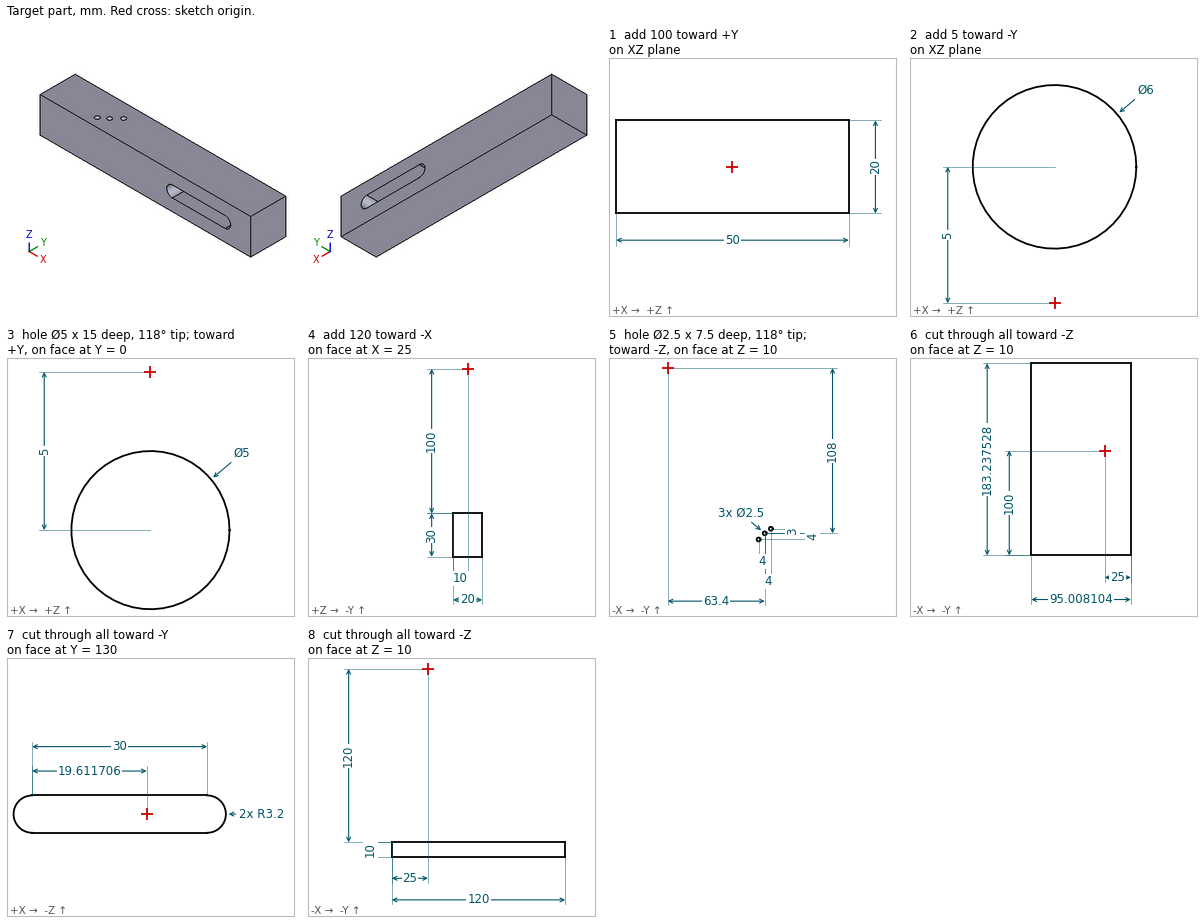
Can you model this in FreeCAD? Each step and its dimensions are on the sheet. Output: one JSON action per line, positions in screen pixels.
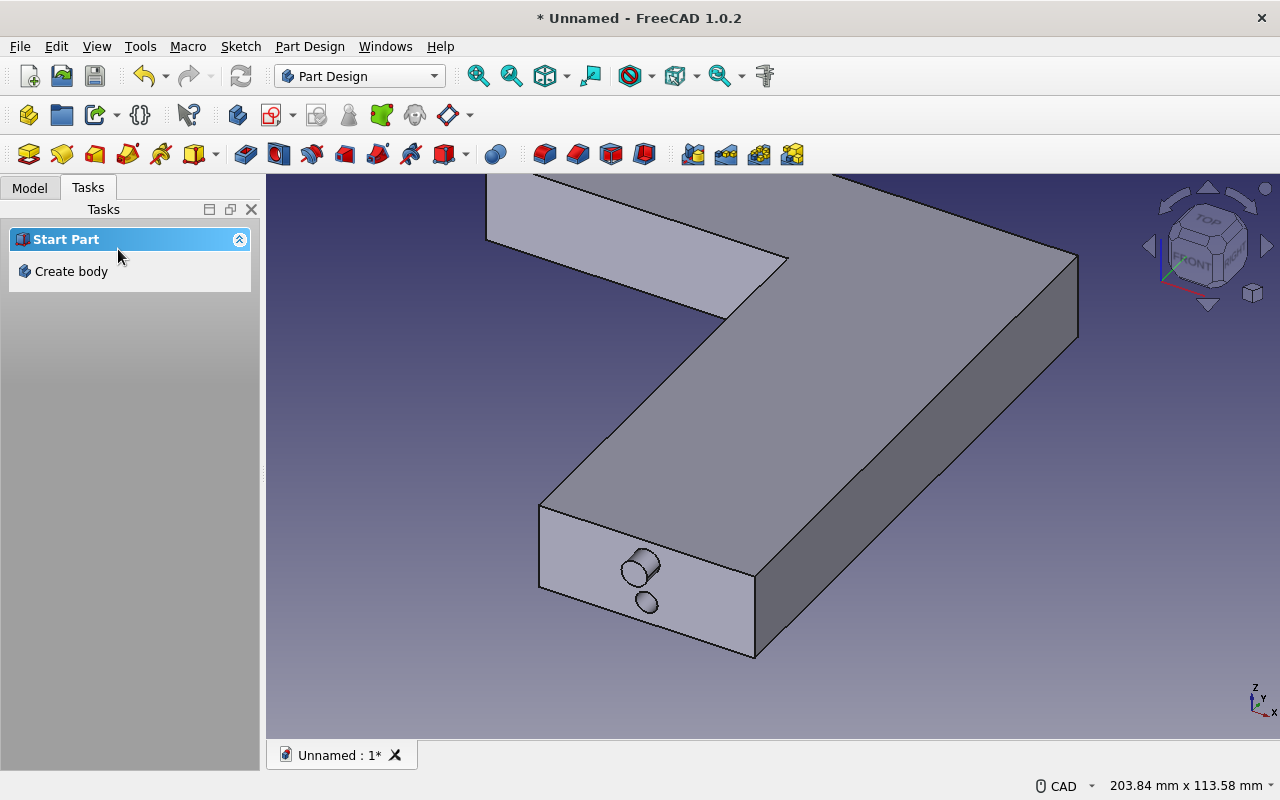
{"action": "left_click", "coordinate": [479, 76]}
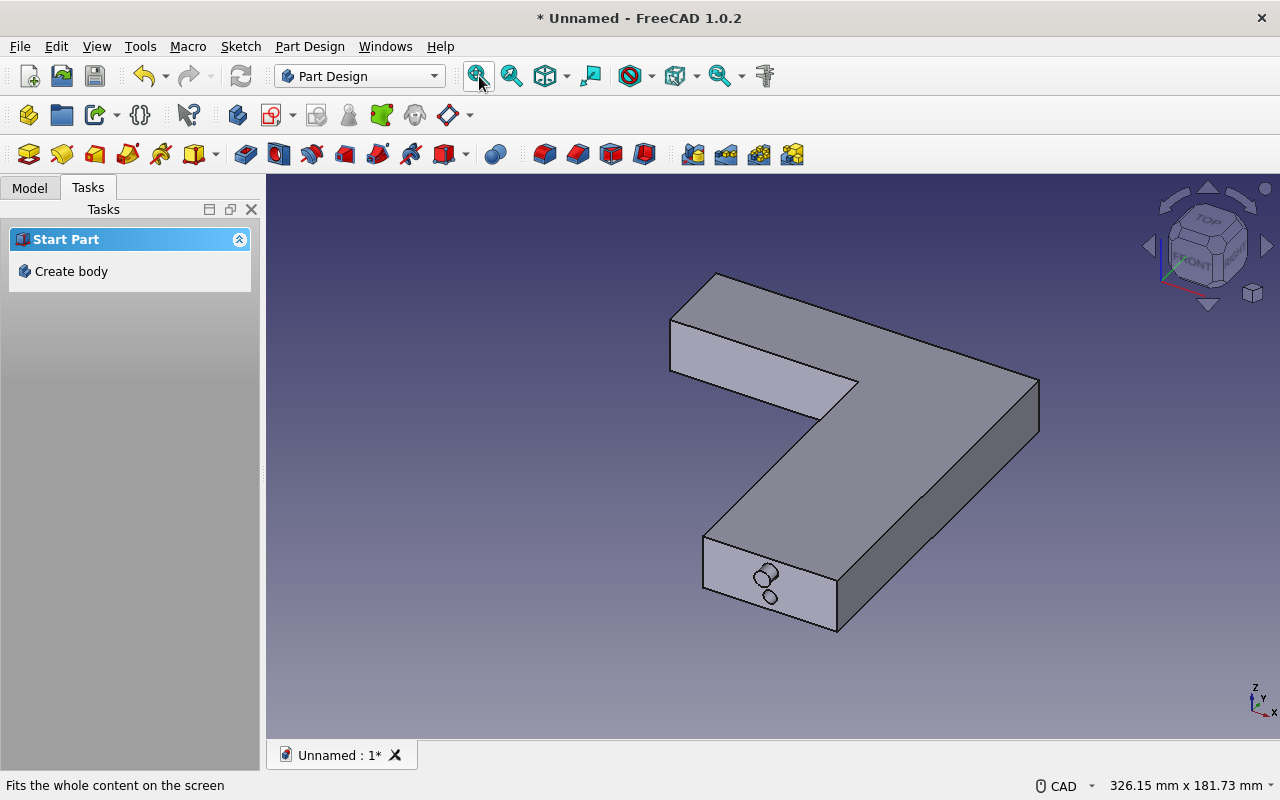
{"action": "left_click", "coordinate": [927, 399]}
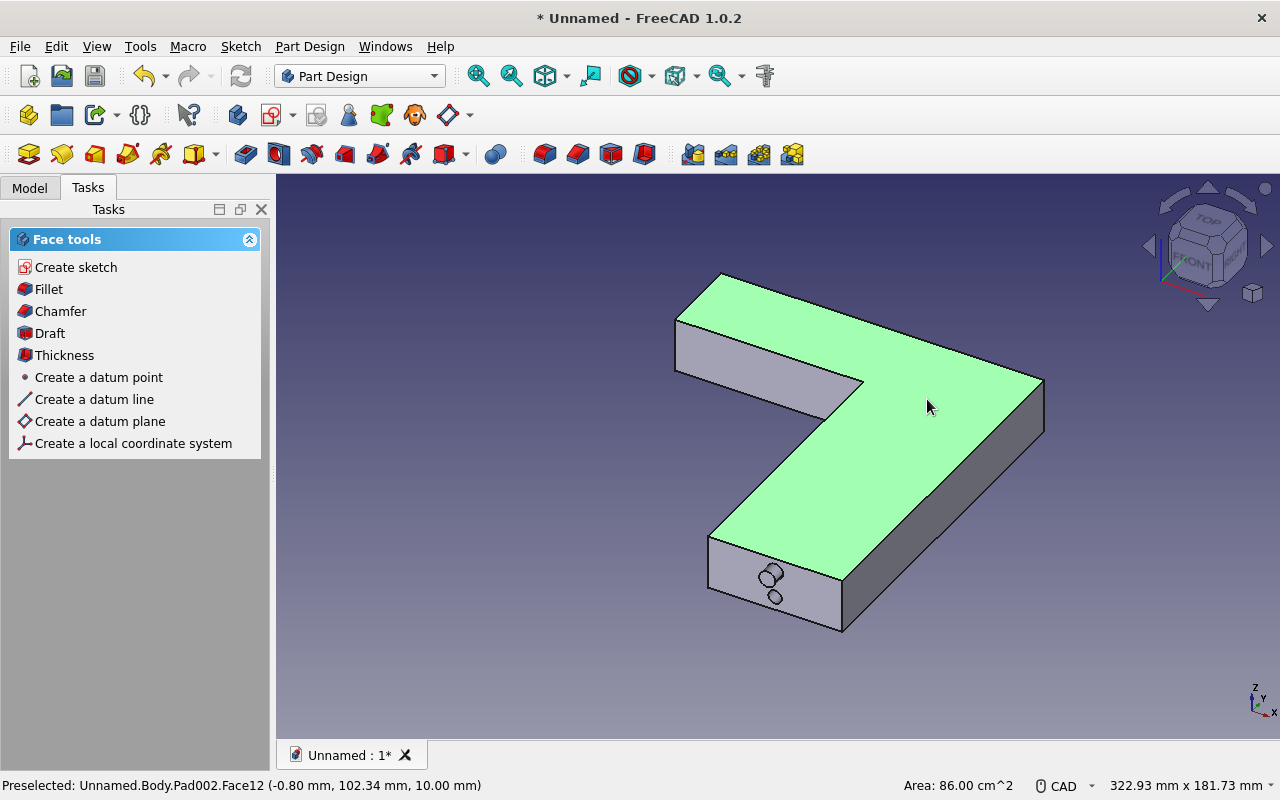
{"action": "left_click", "coordinate": [270, 116]}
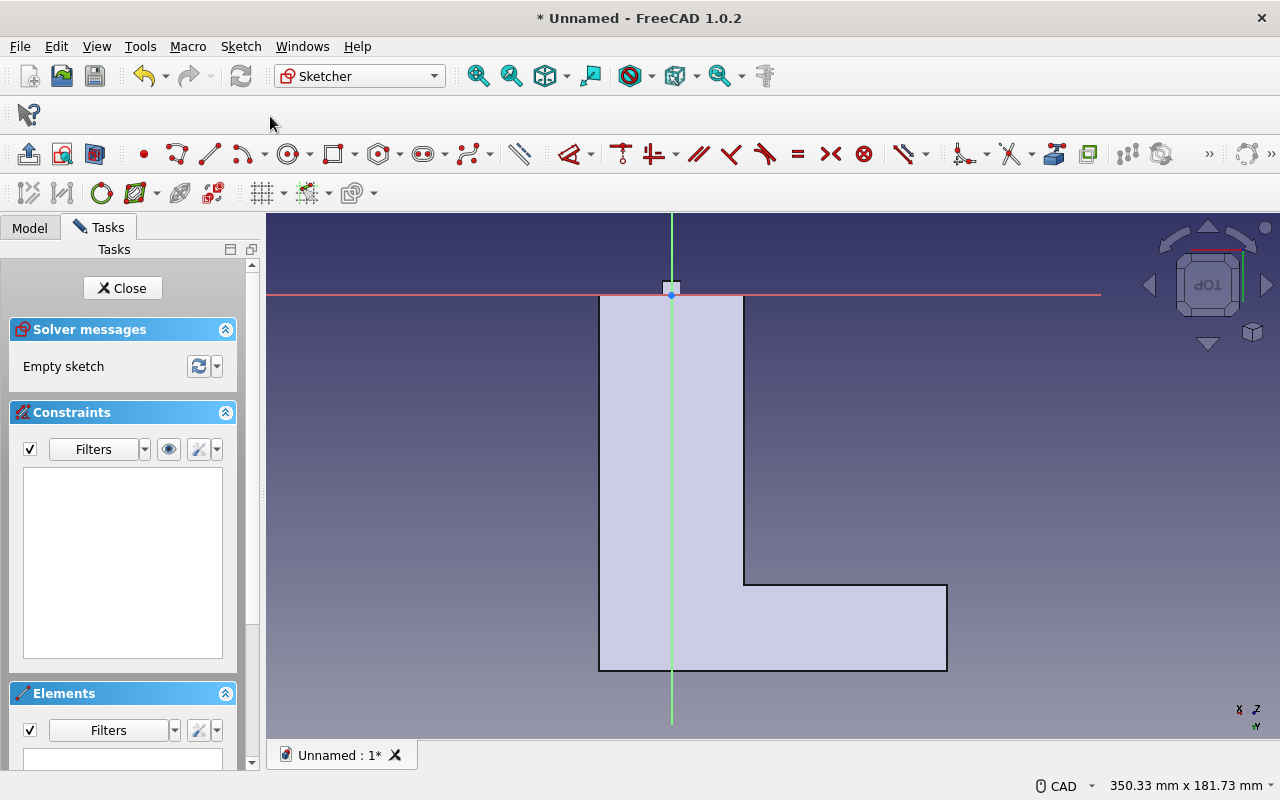
{"action": "scroll", "coordinate": [870, 622], "scroll_direction": "up", "scroll_amount": 12}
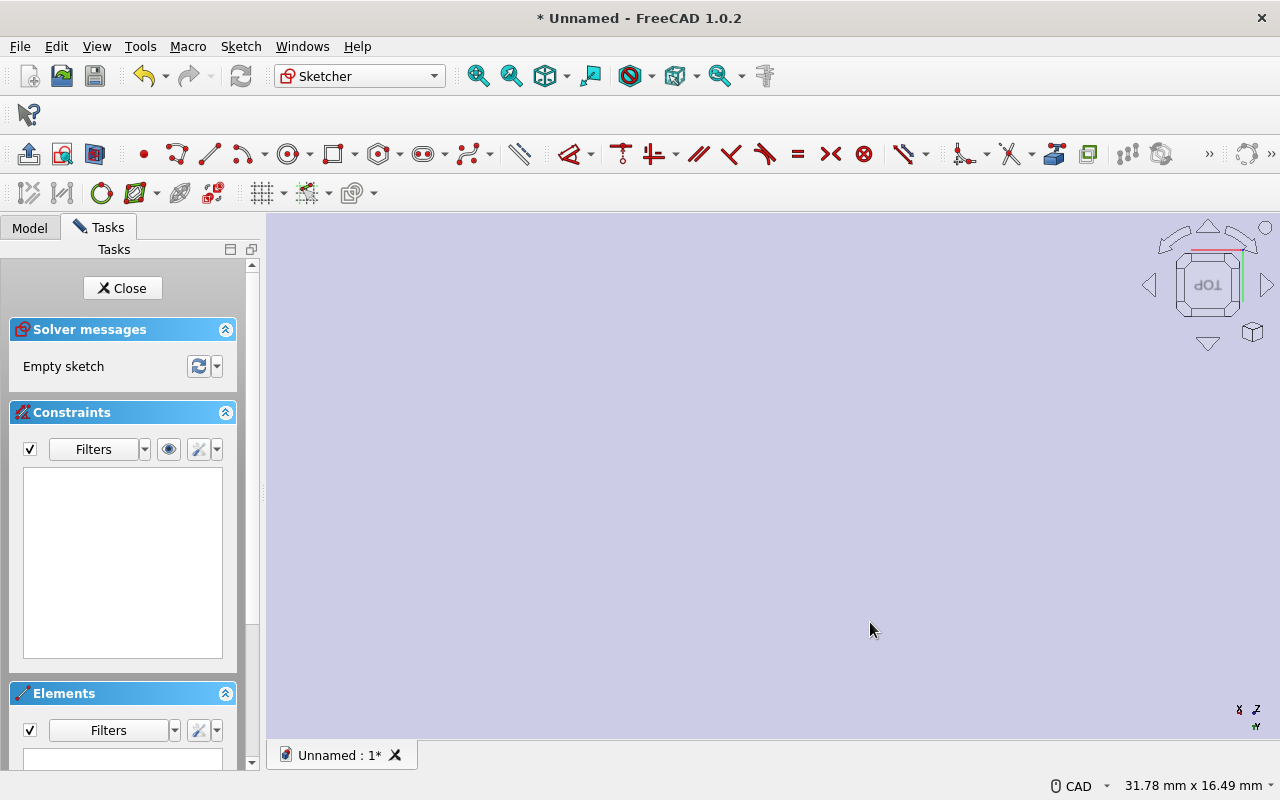
{"action": "left_click", "coordinate": [288, 154]}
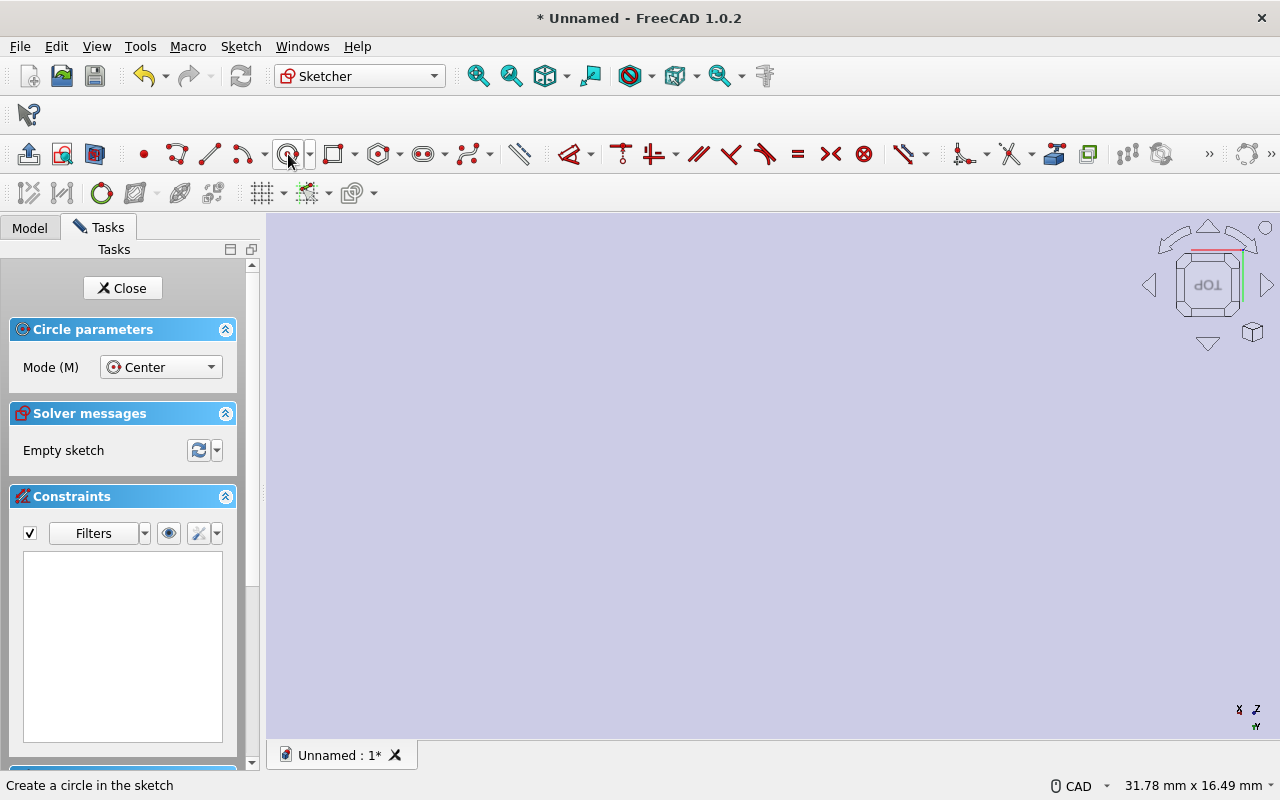
{"action": "left_click", "coordinate": [701, 457]}
{"action": "left_click", "coordinate": [729, 428]}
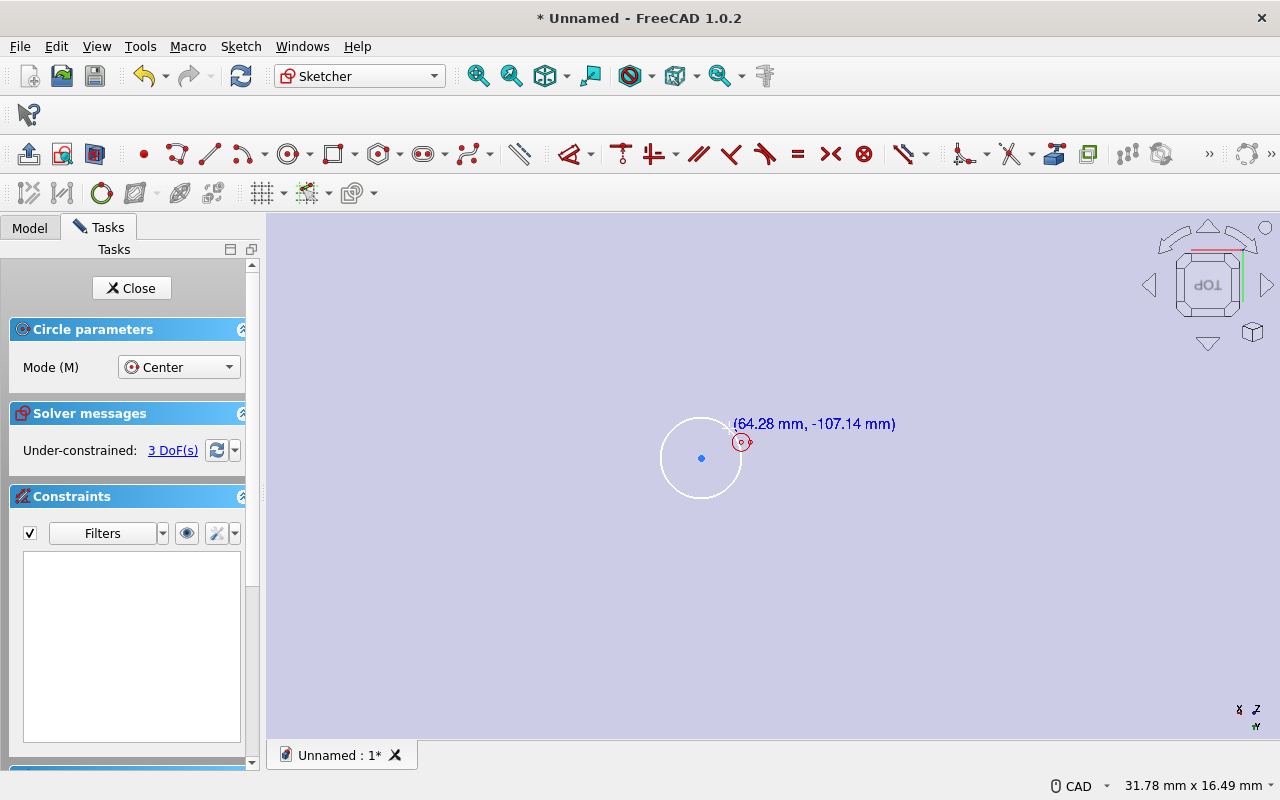
{"action": "left_click", "coordinate": [573, 584]}
{"action": "left_click", "coordinate": [601, 556]}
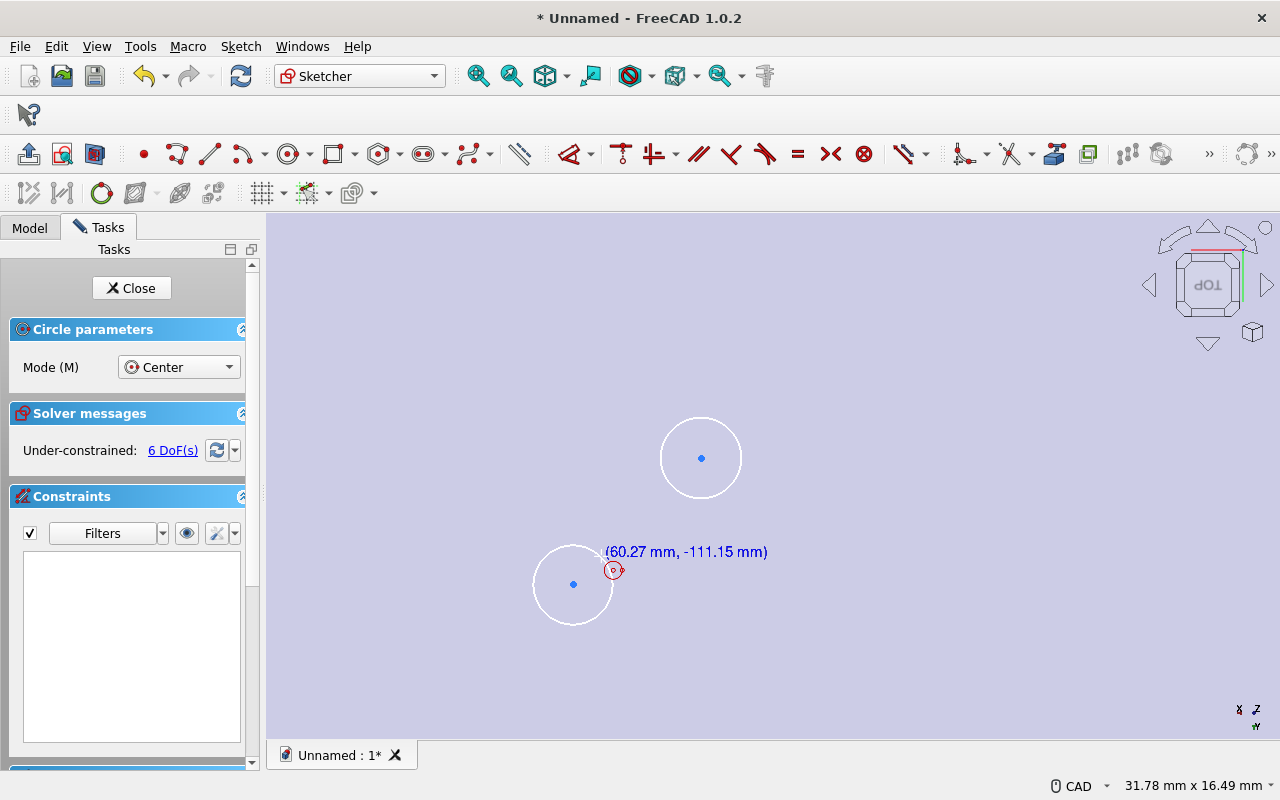
{"action": "left_click", "coordinate": [829, 361]}
{"action": "left_click", "coordinate": [857, 333]}
{"action": "key", "text": "Escape"}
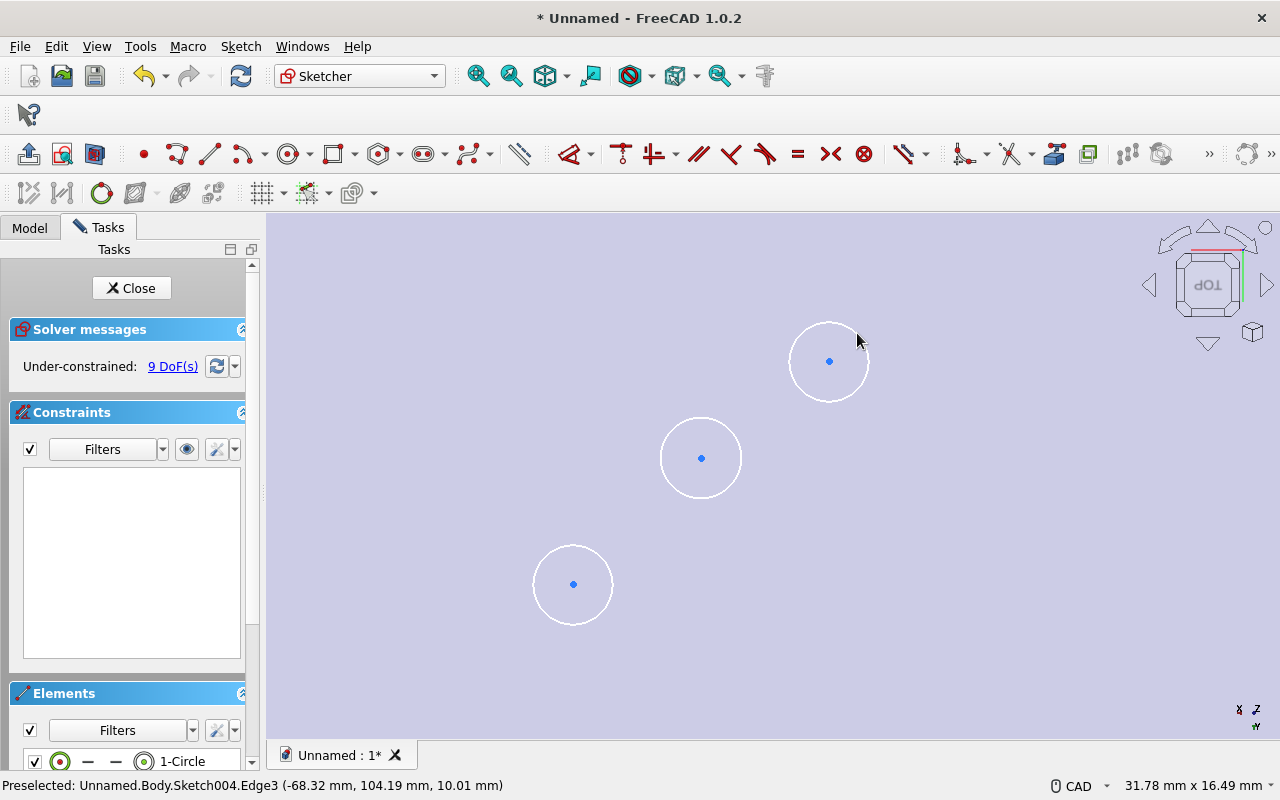
{"action": "left_click", "coordinate": [729, 429]}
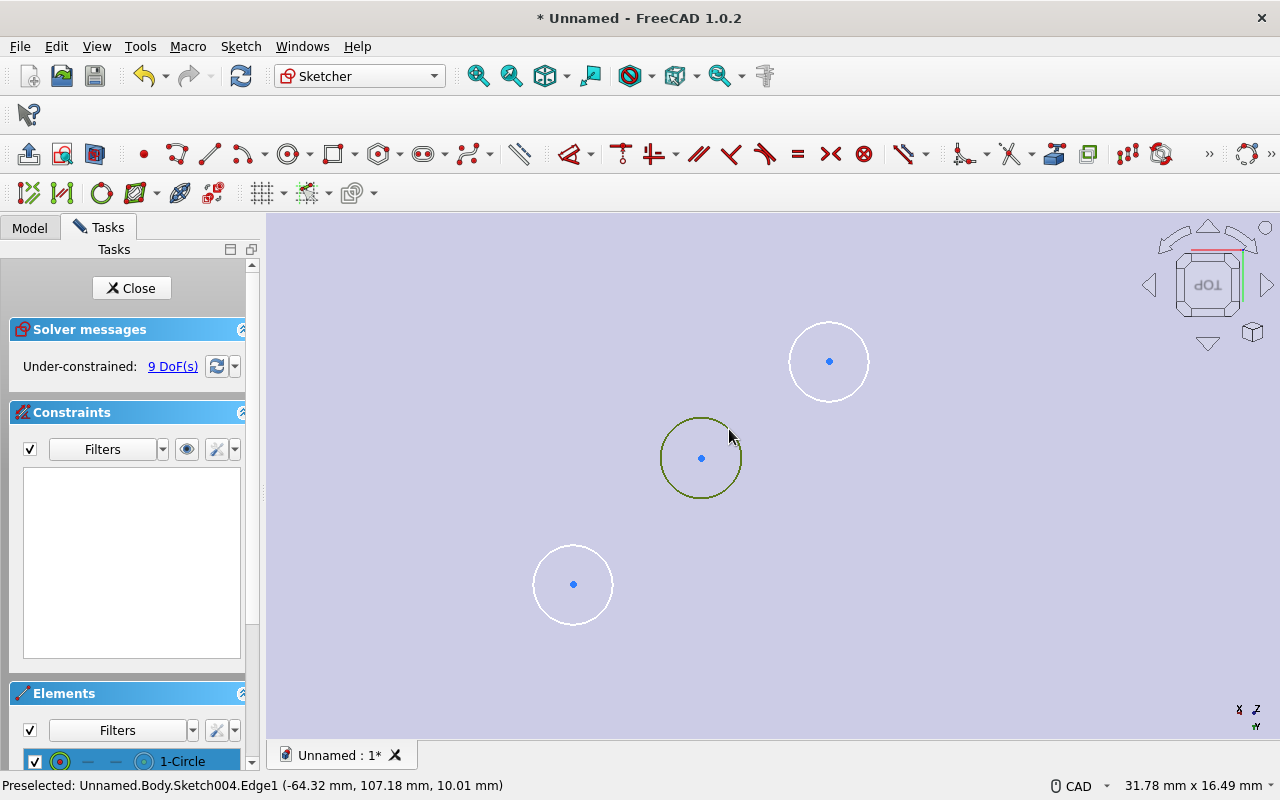
{"action": "left_click", "coordinate": [601, 557]}